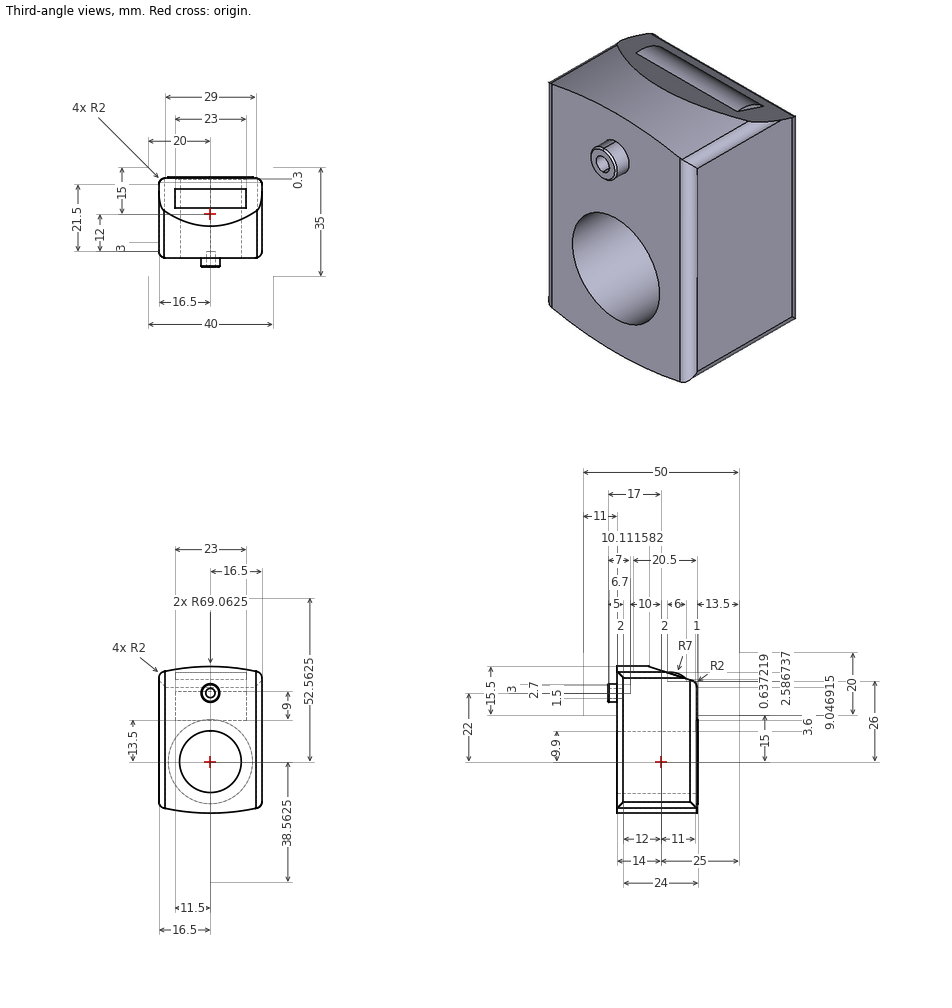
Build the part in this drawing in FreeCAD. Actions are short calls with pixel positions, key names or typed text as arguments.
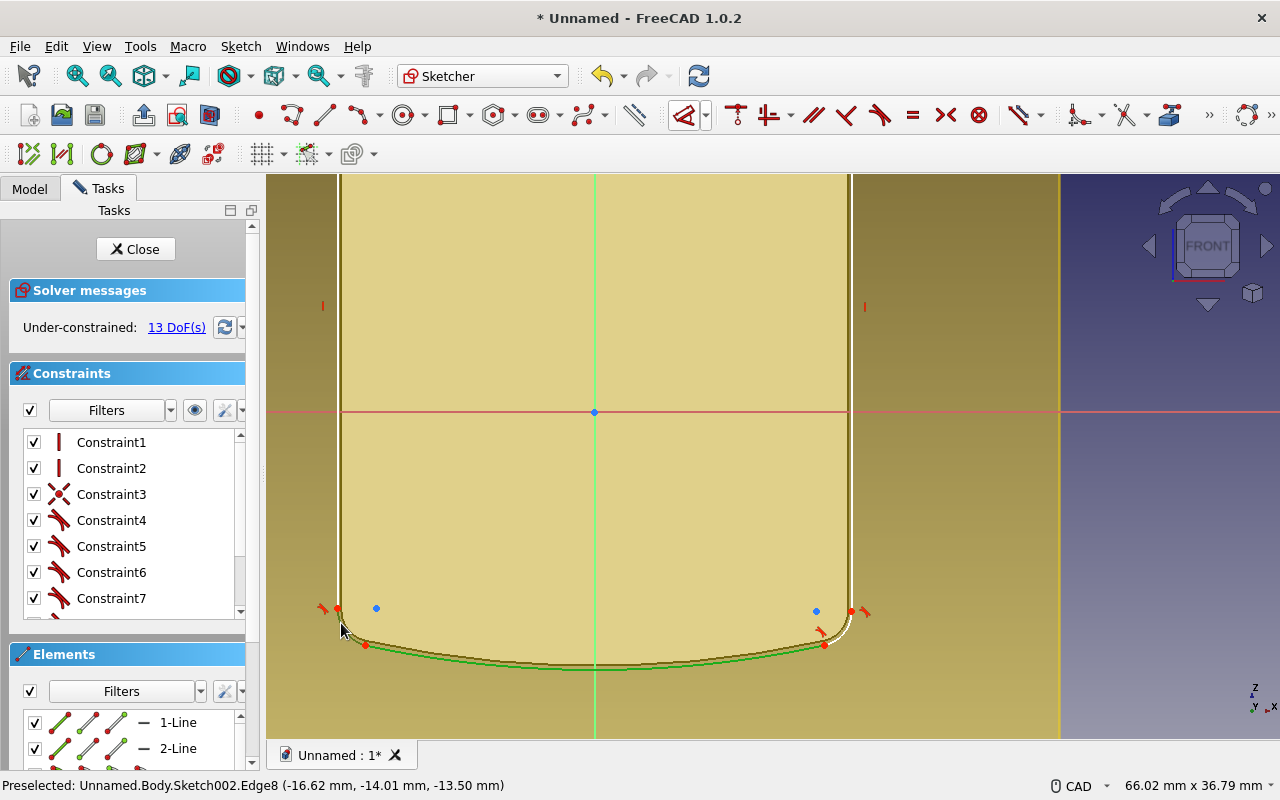
click(880, 116)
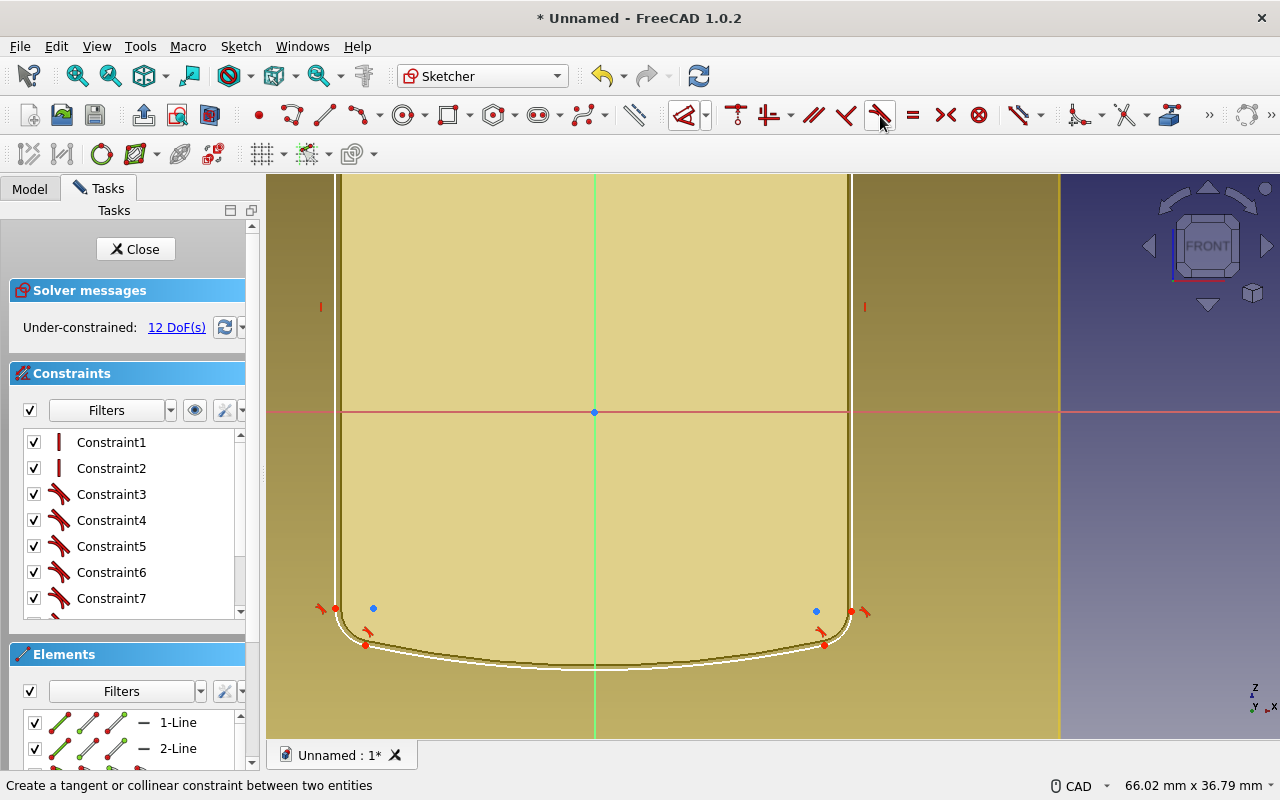
scroll(838, 641, down, 3)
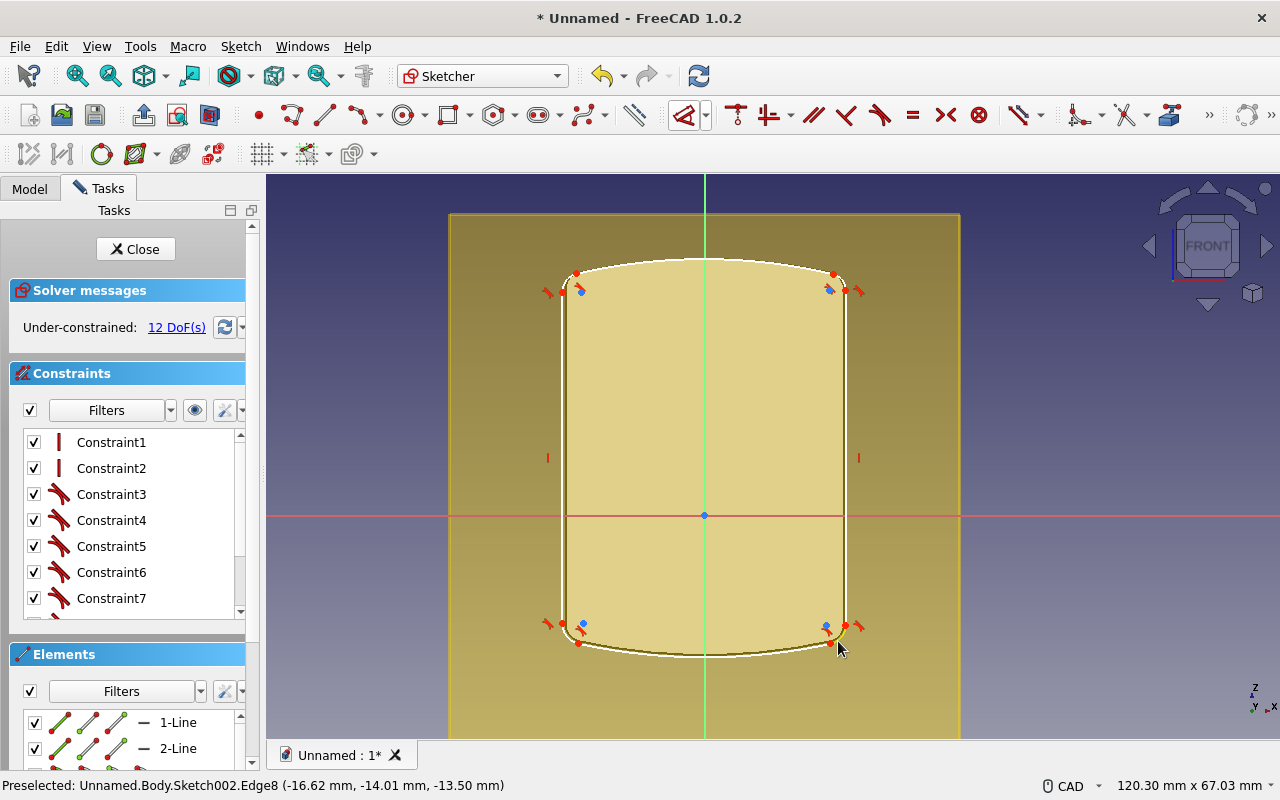
scroll(570, 277, up, 4)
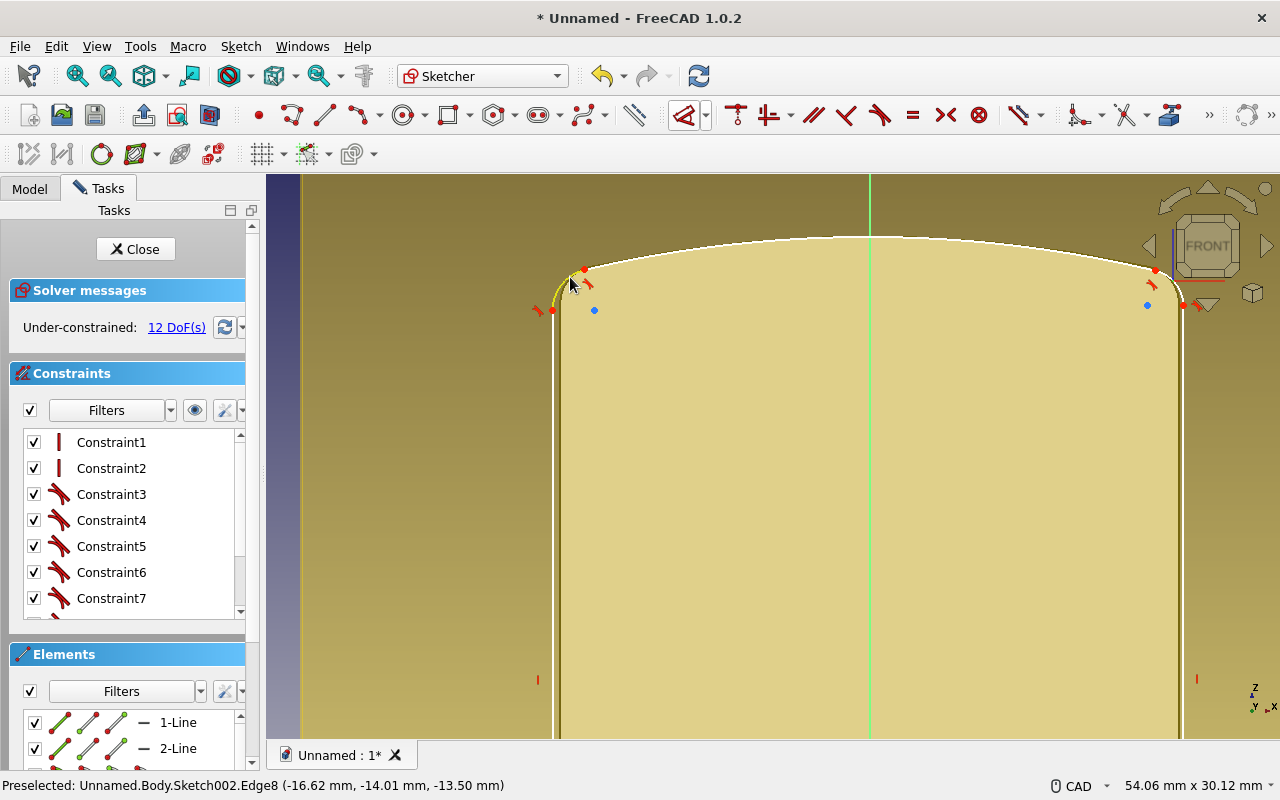
click(570, 277)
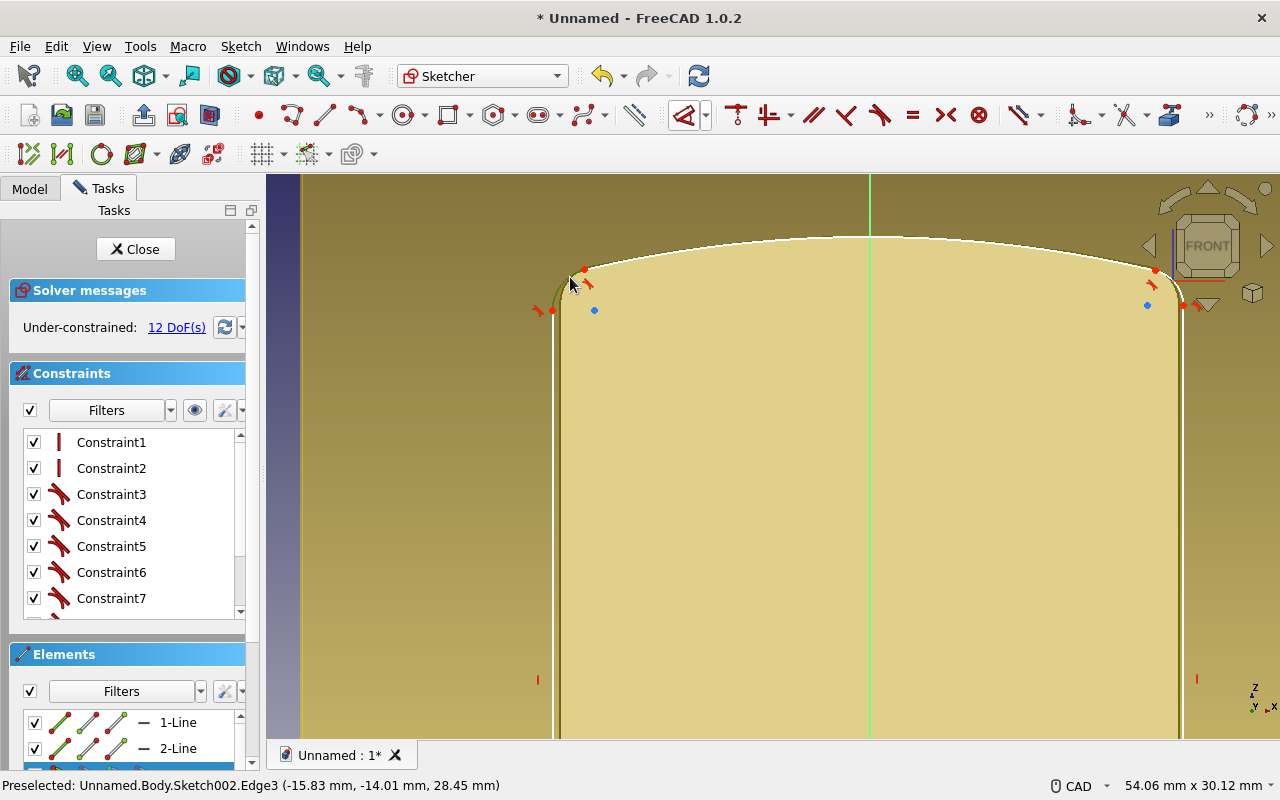
scroll(570, 276, down, 4)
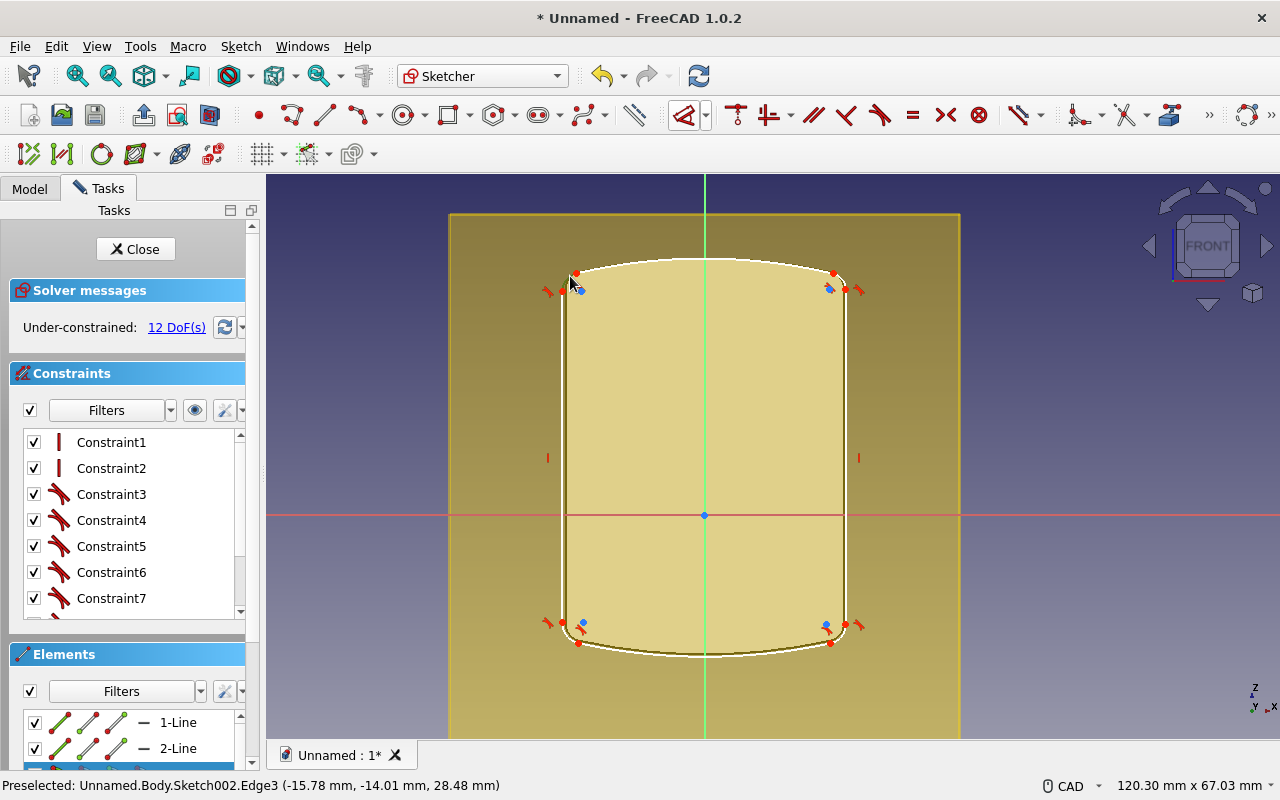
scroll(844, 283, up, 4)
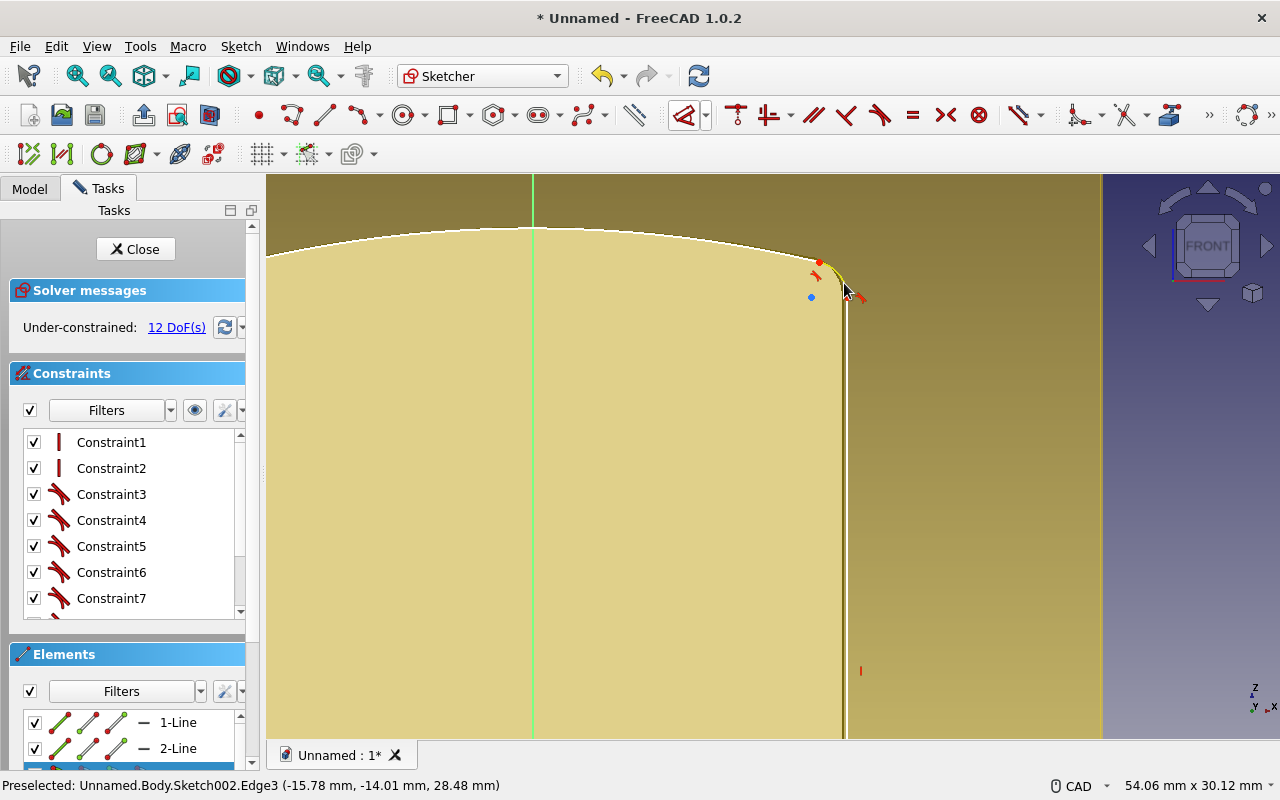
click(844, 283)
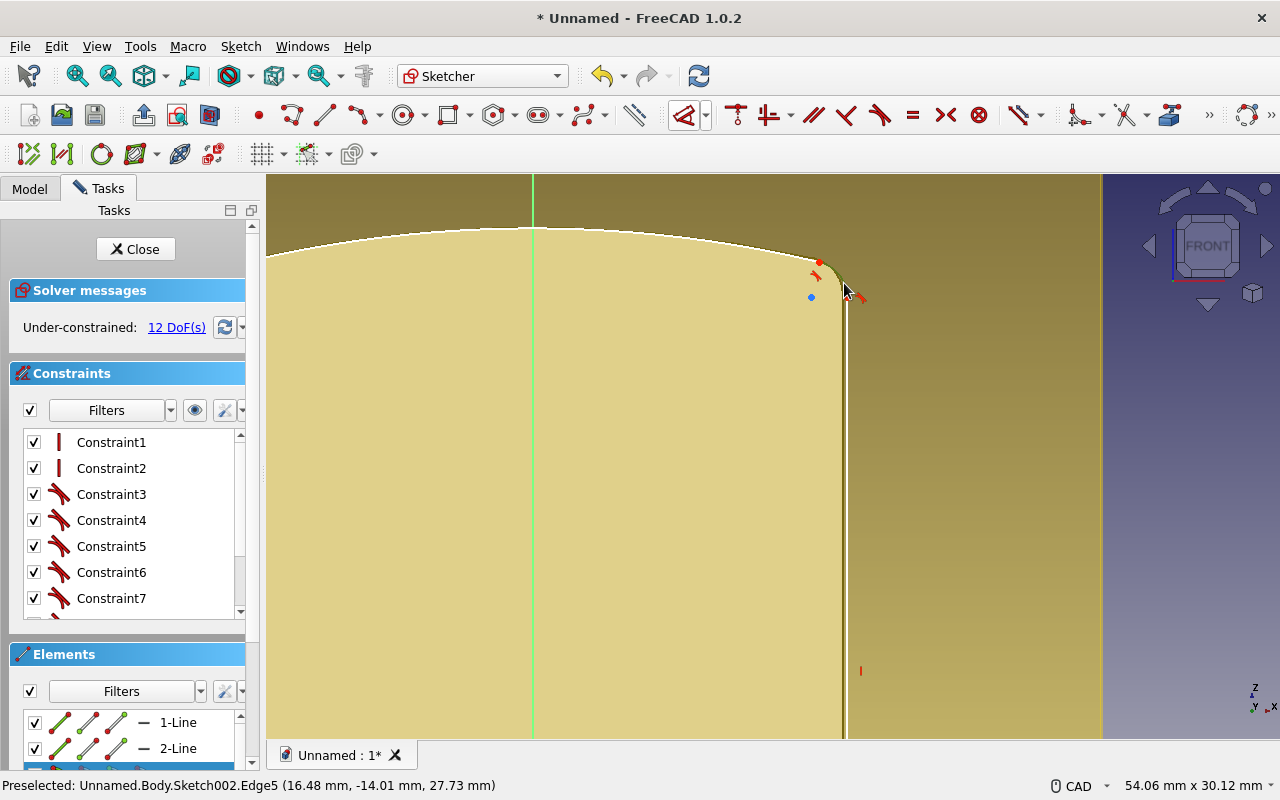
scroll(844, 283, down, 4)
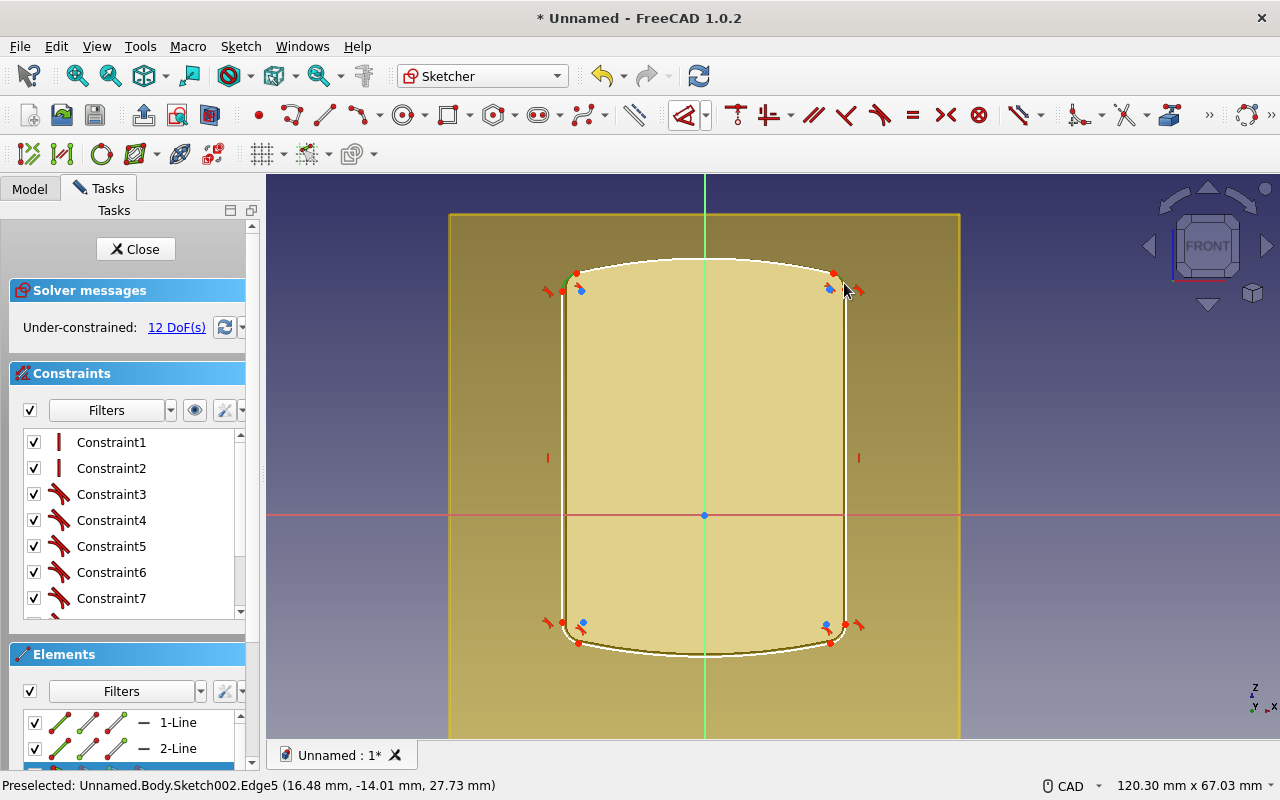
scroll(838, 640, up, 3)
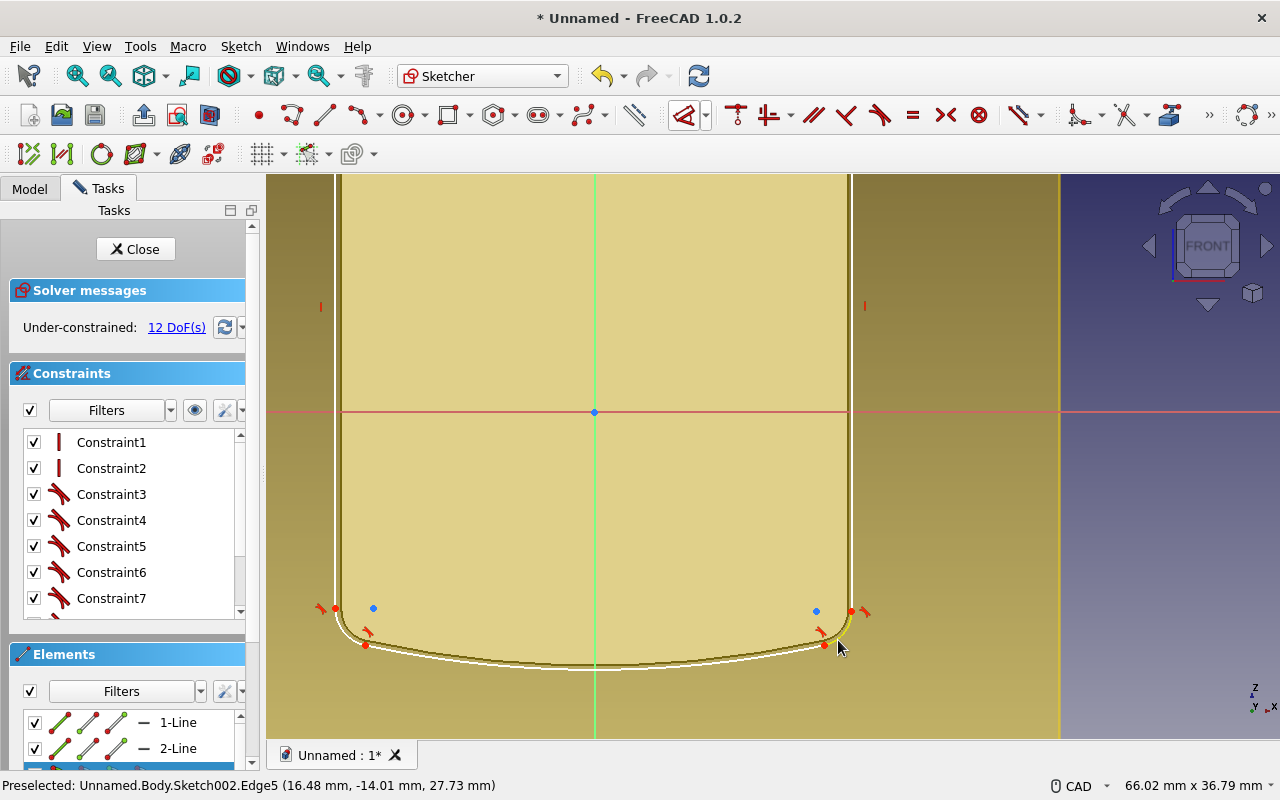
click(837, 640)